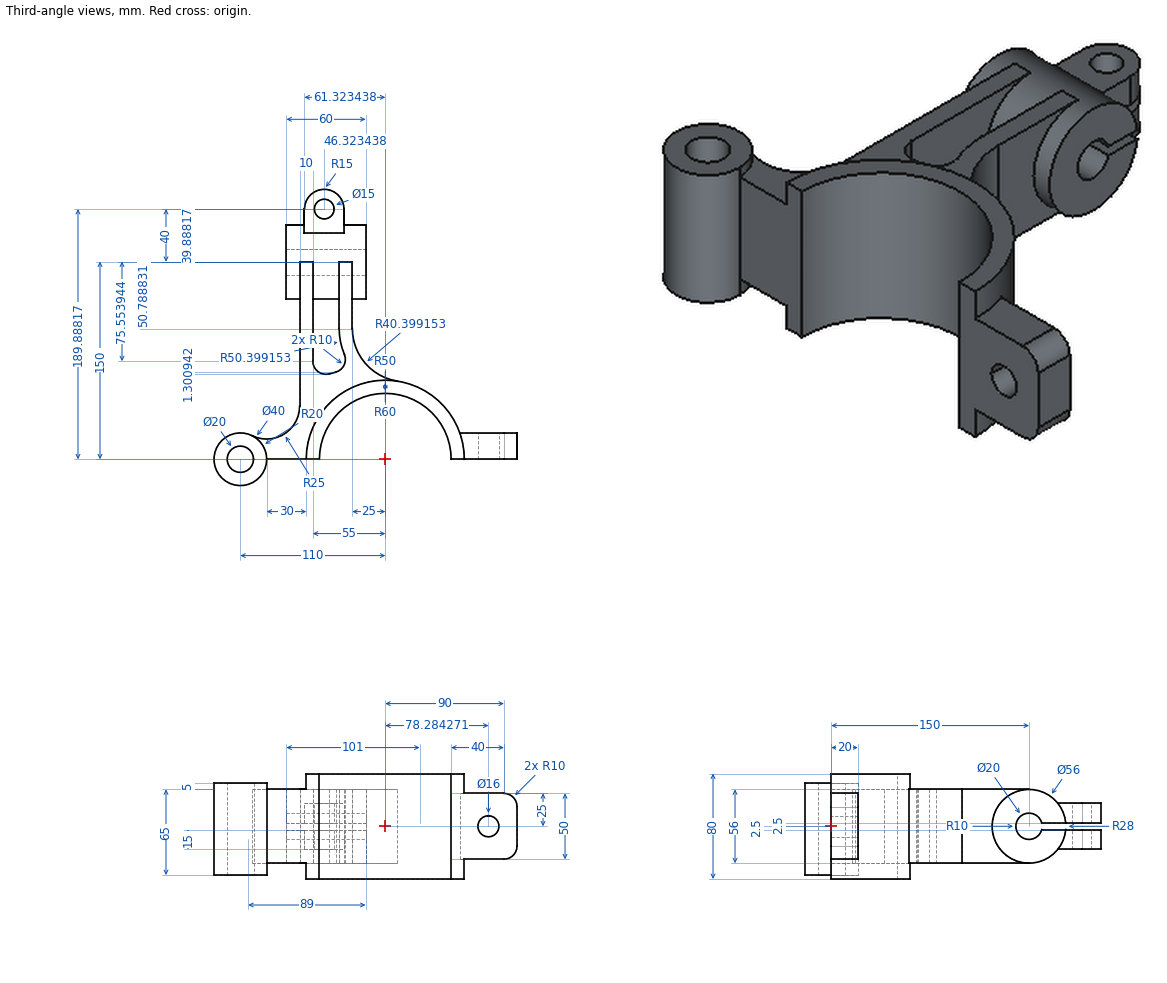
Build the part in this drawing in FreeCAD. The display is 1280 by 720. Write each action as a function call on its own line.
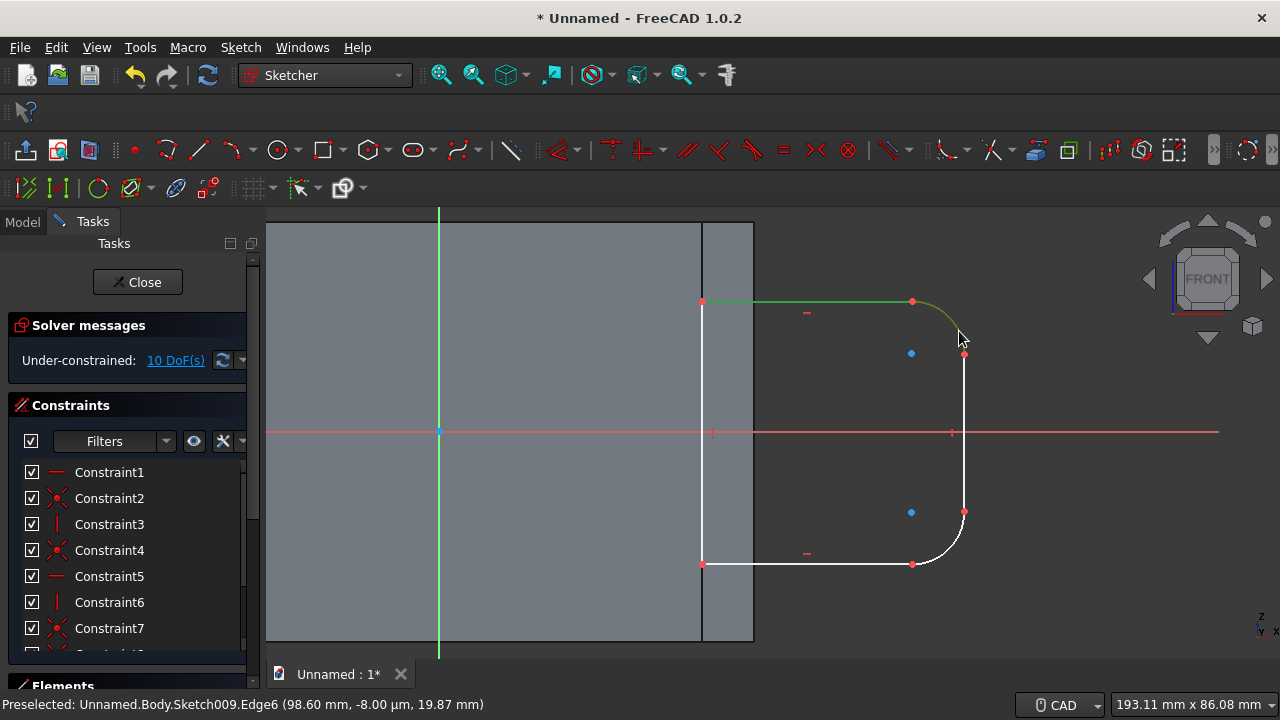
click(752, 150)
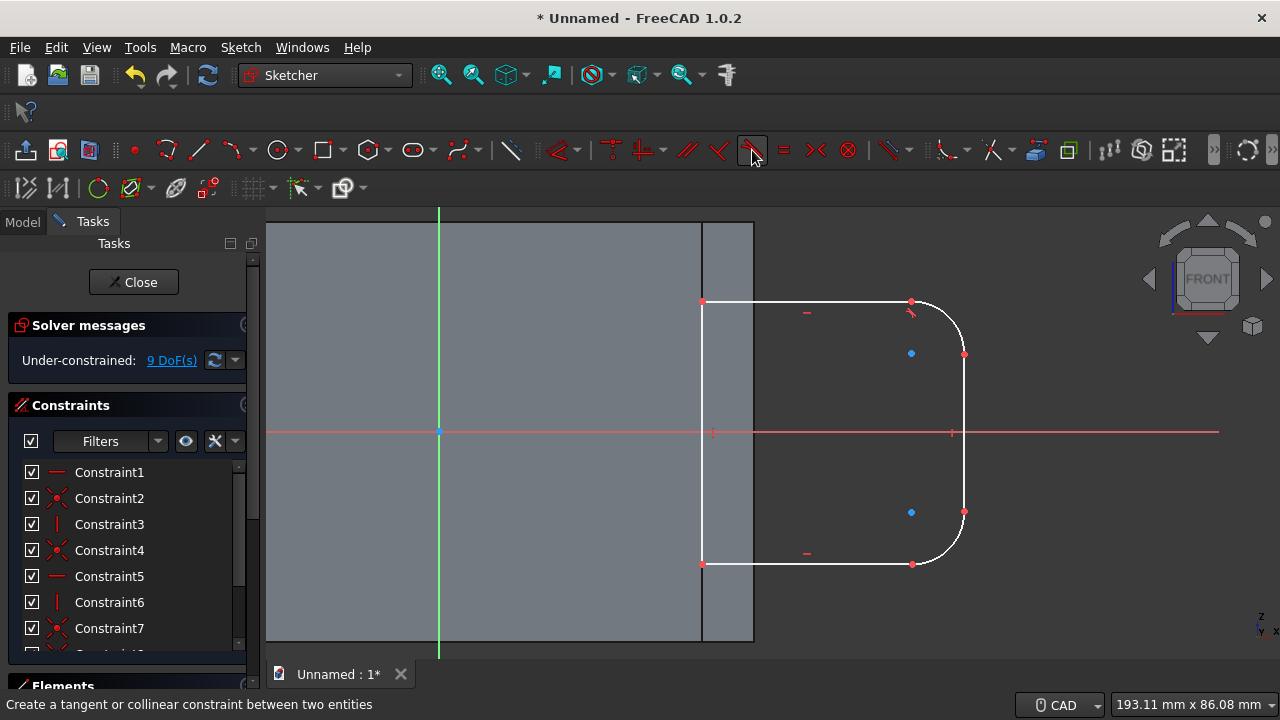
click(765, 564)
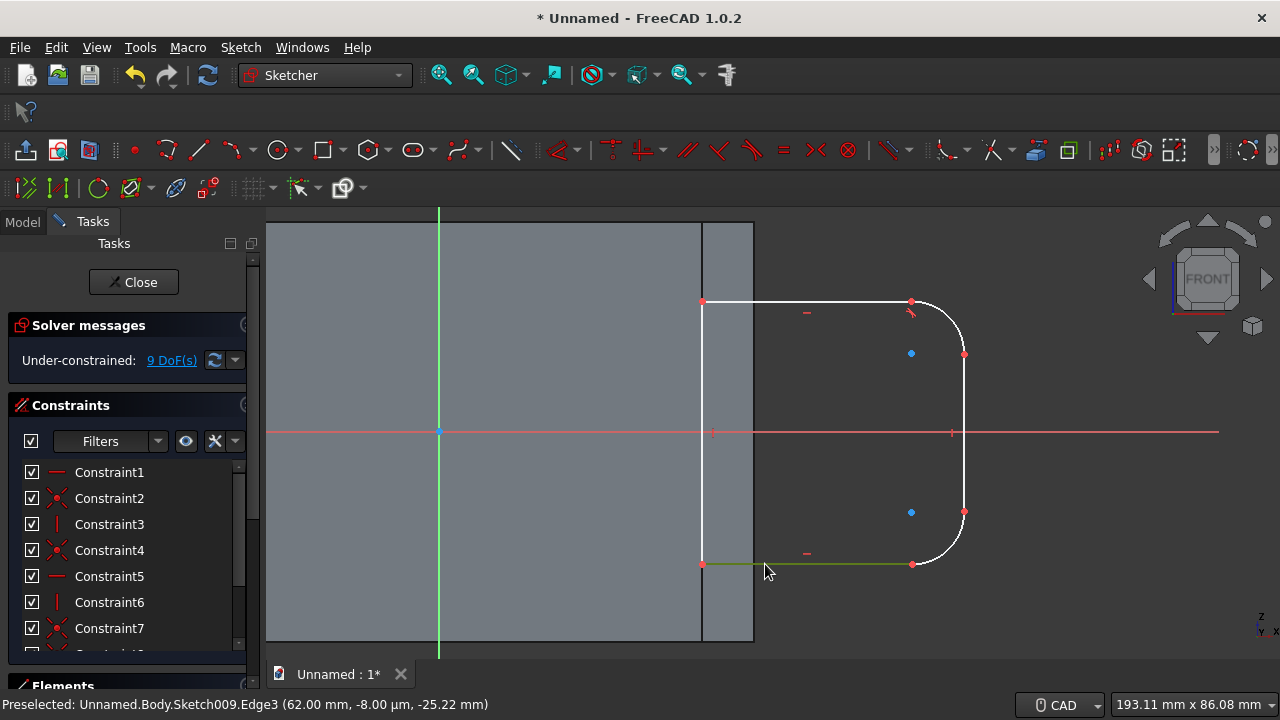
click(936, 559)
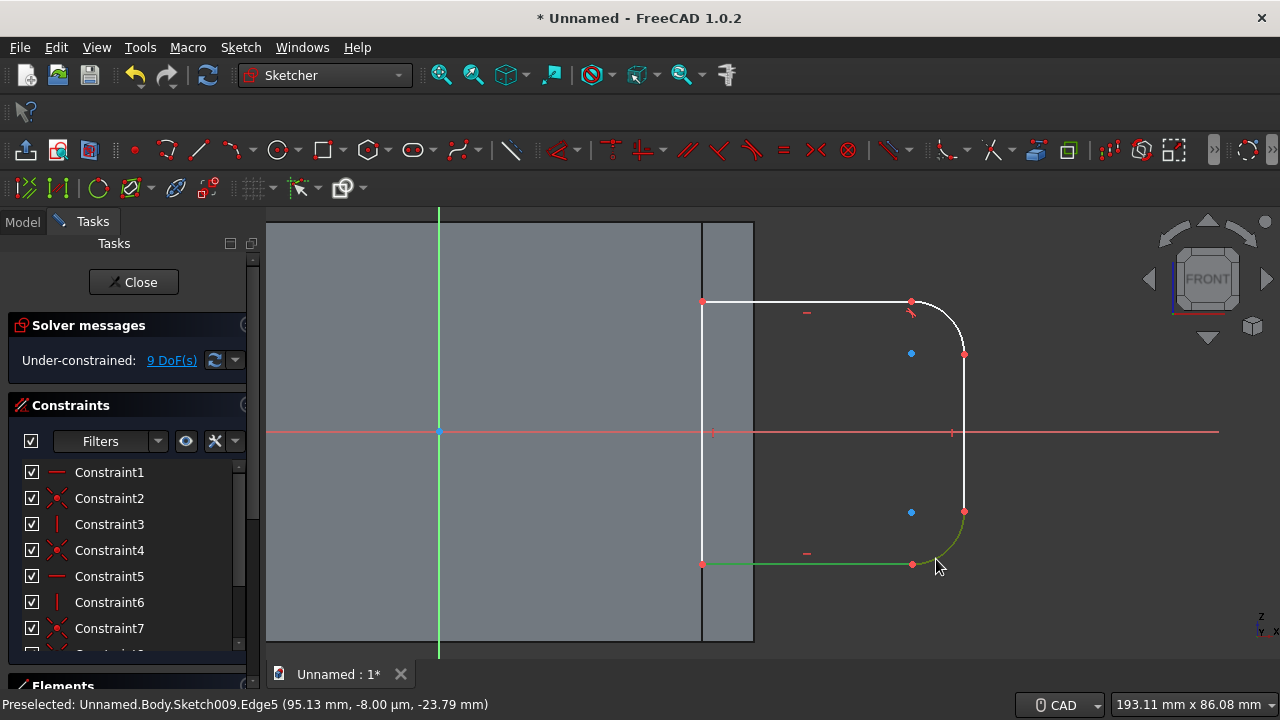
key(t)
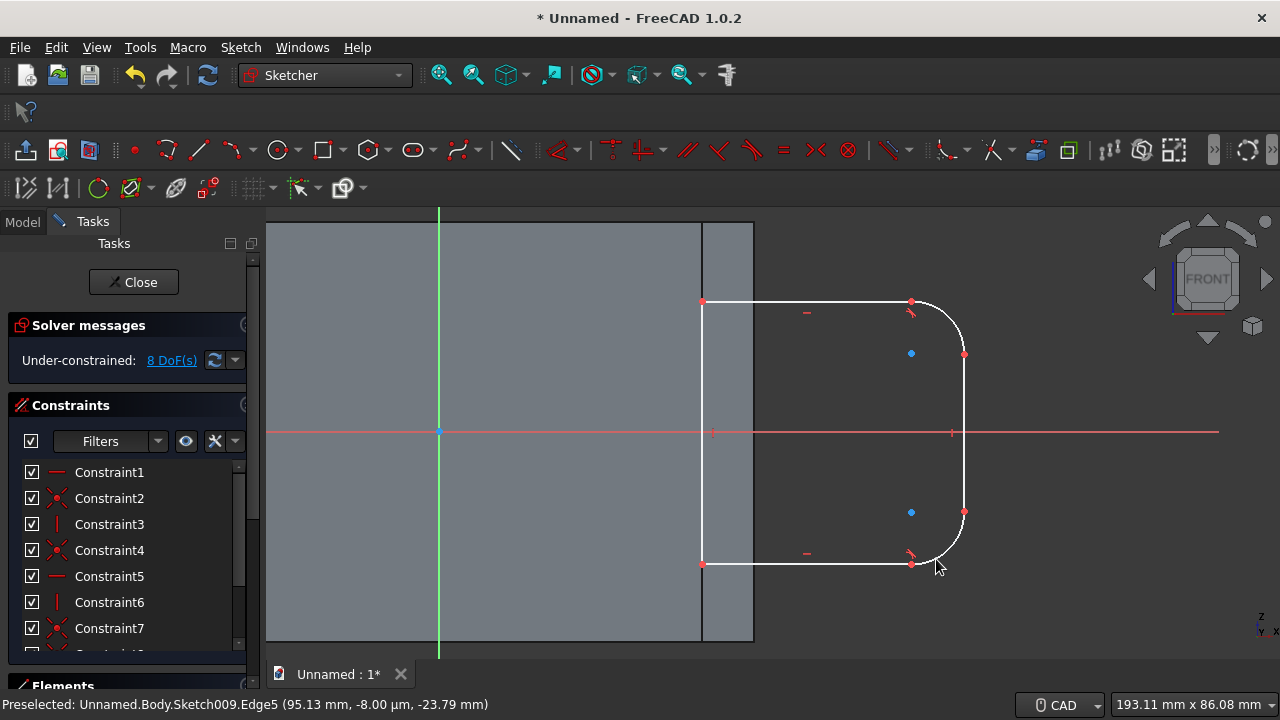
click(964, 464)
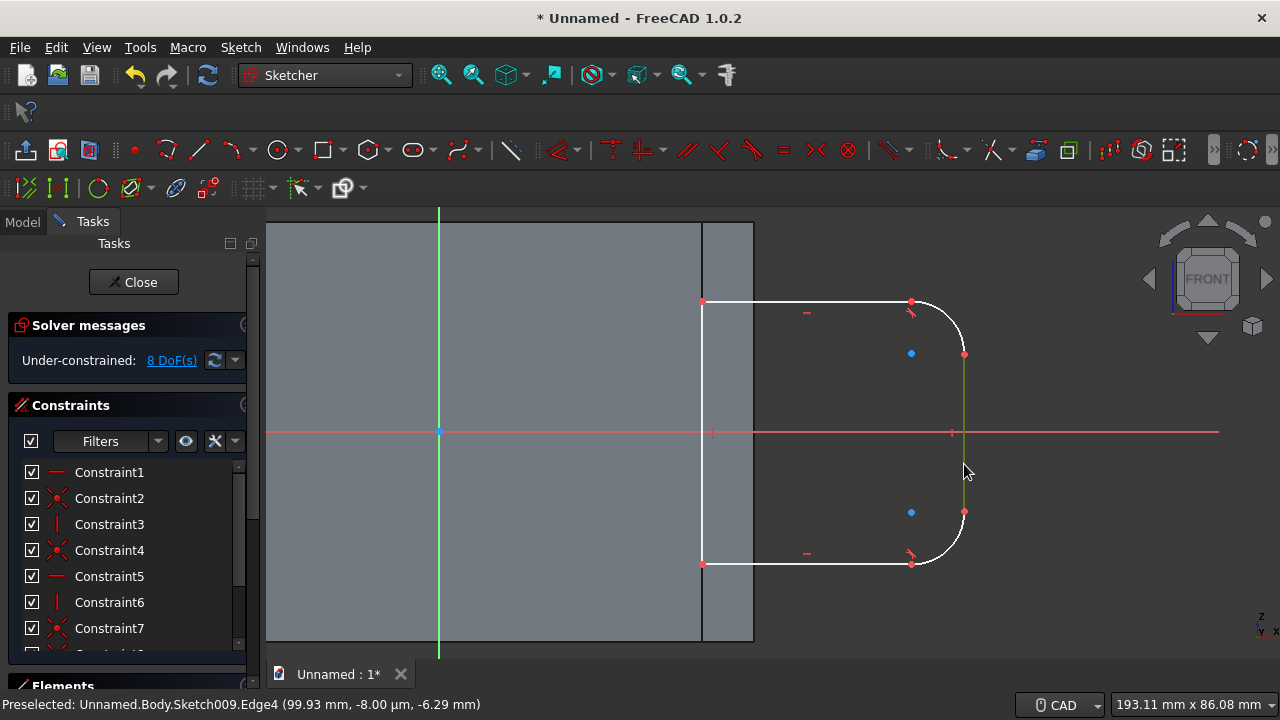
click(936, 559)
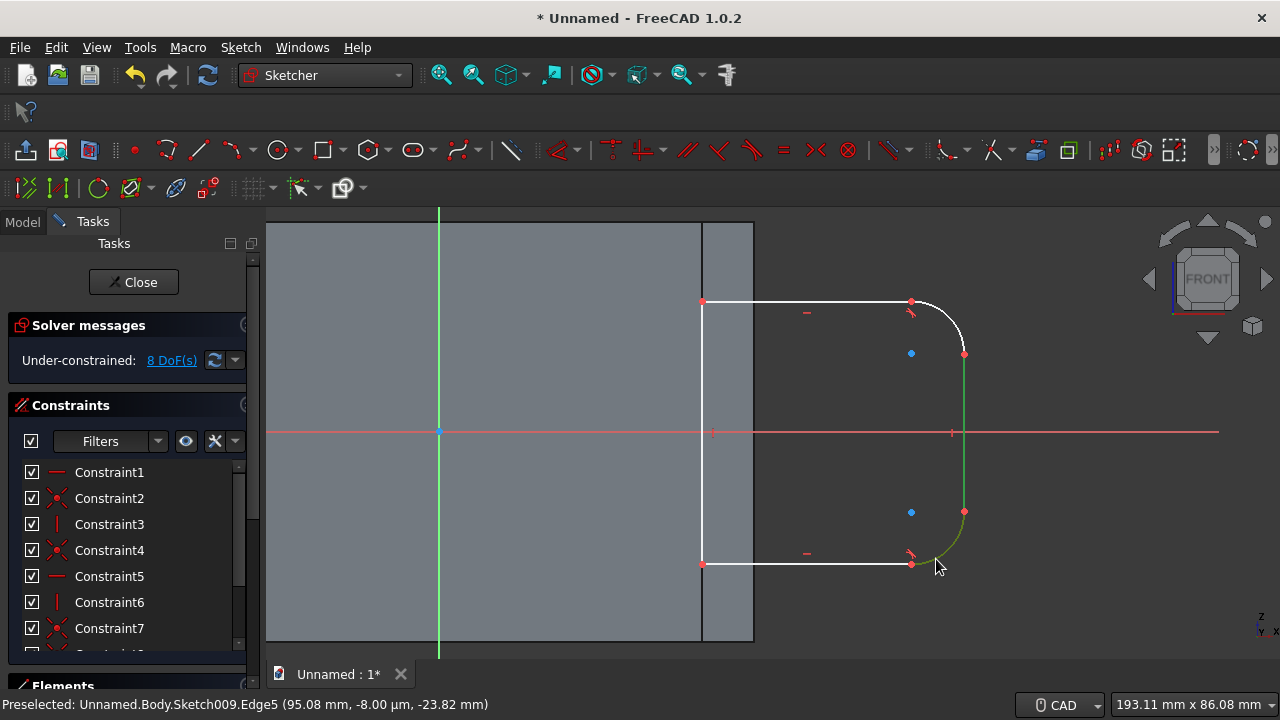
click(752, 150)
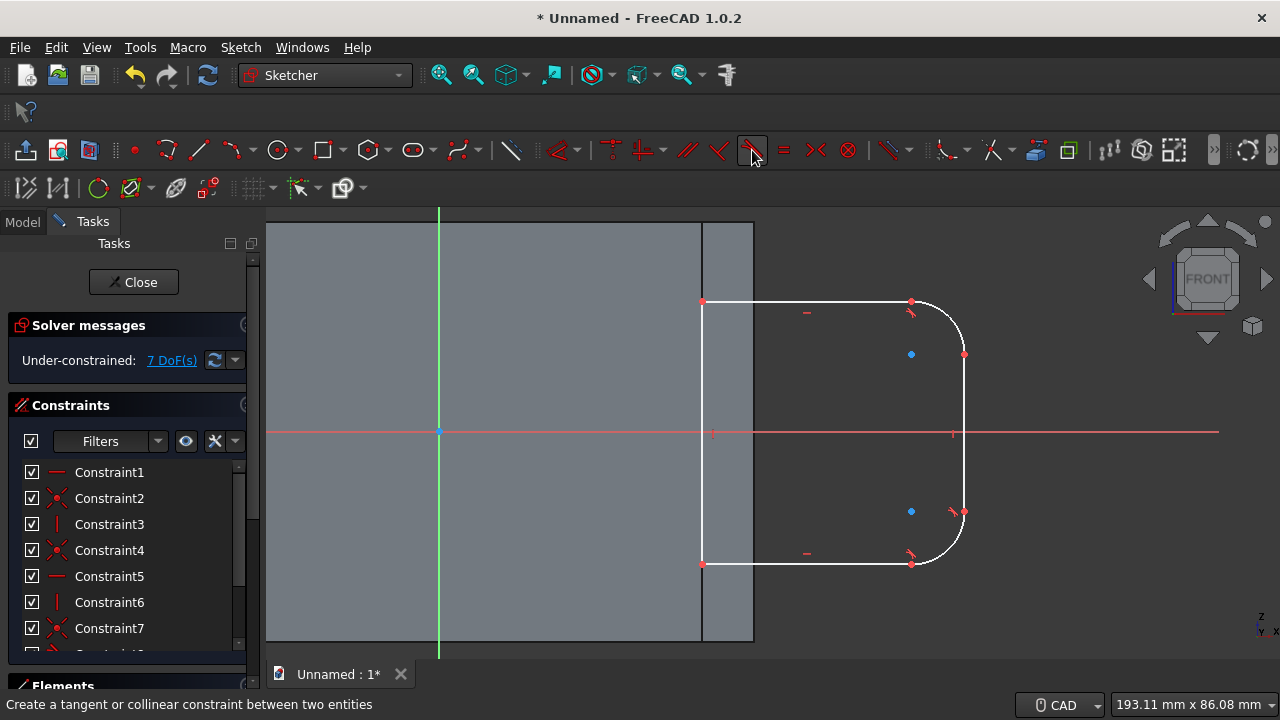
click(964, 464)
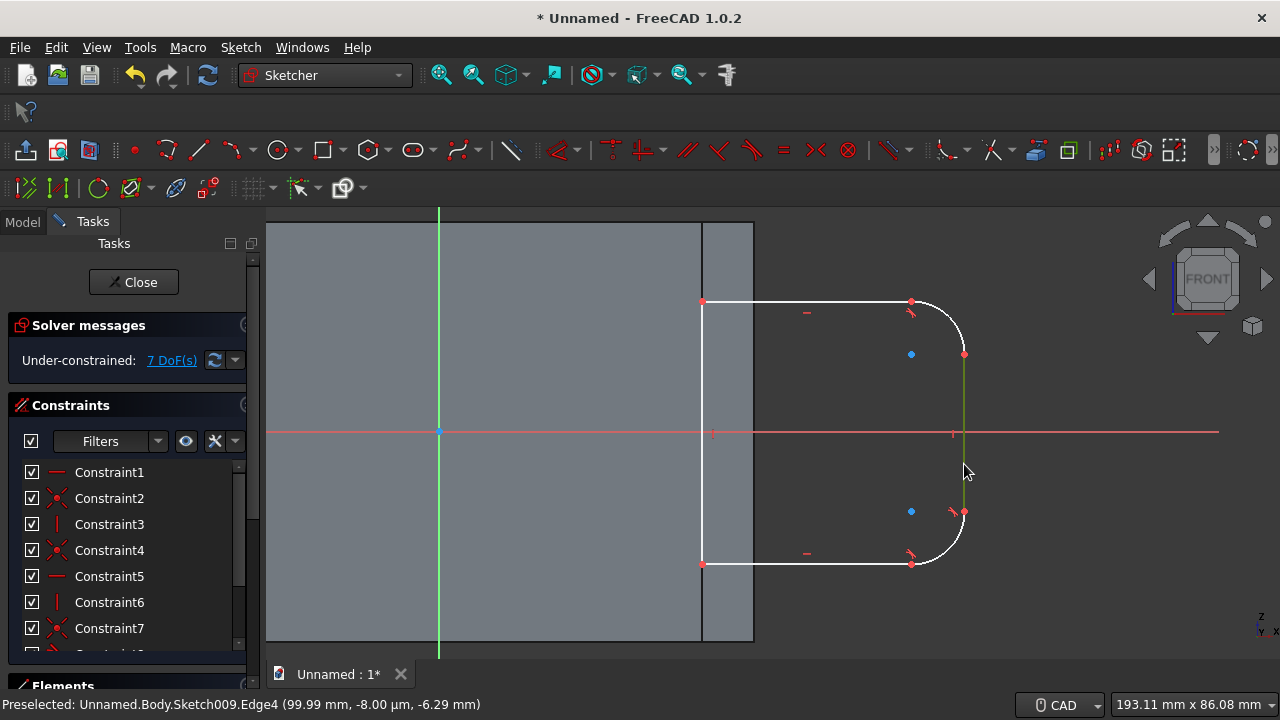
click(959, 330)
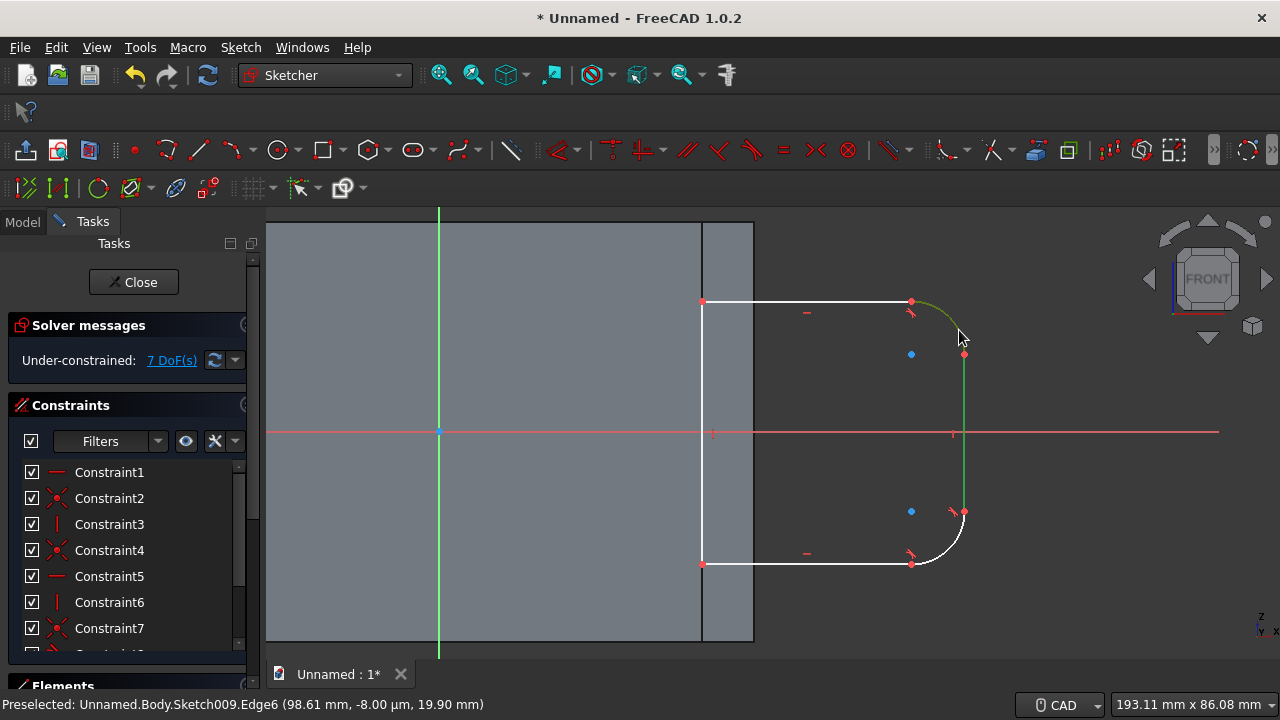
key(t)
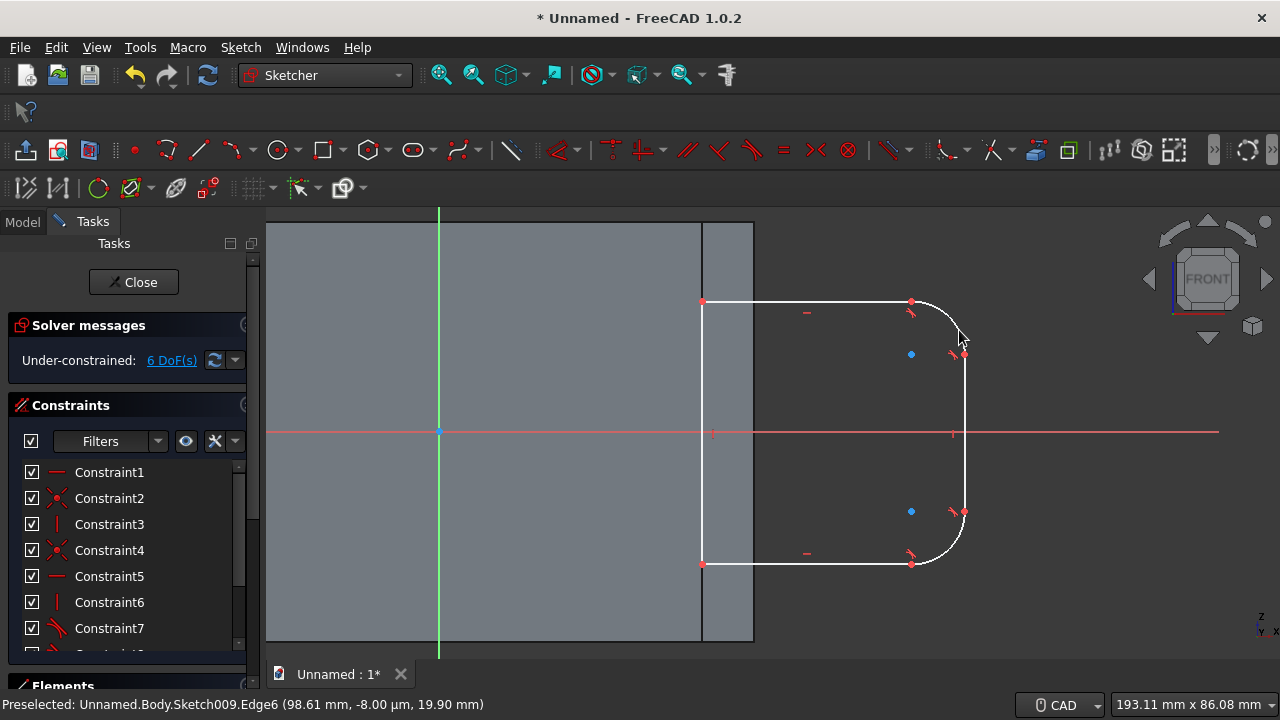
click(936, 559)